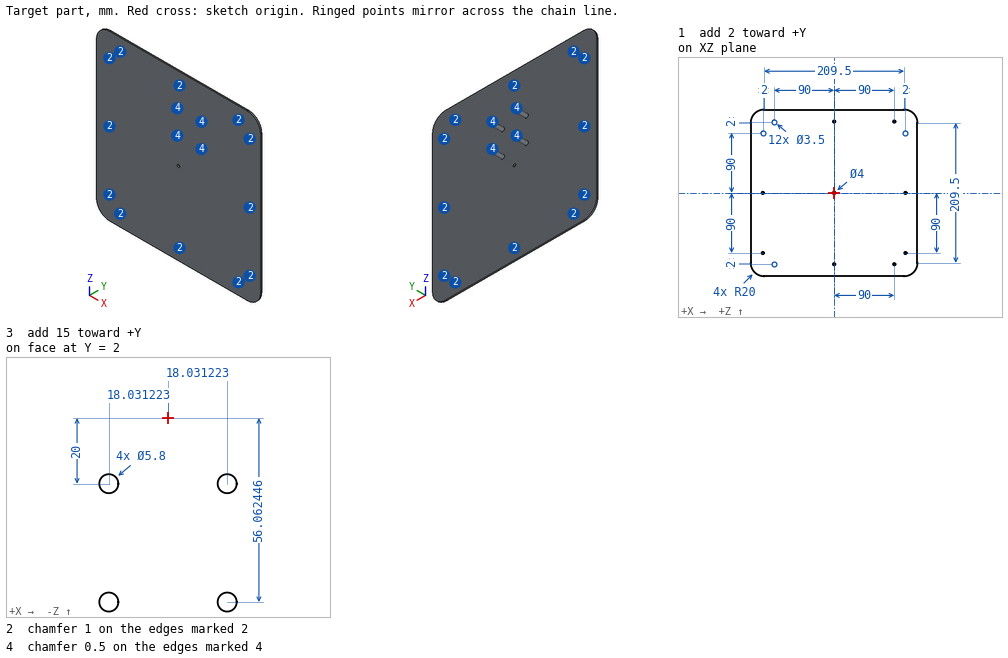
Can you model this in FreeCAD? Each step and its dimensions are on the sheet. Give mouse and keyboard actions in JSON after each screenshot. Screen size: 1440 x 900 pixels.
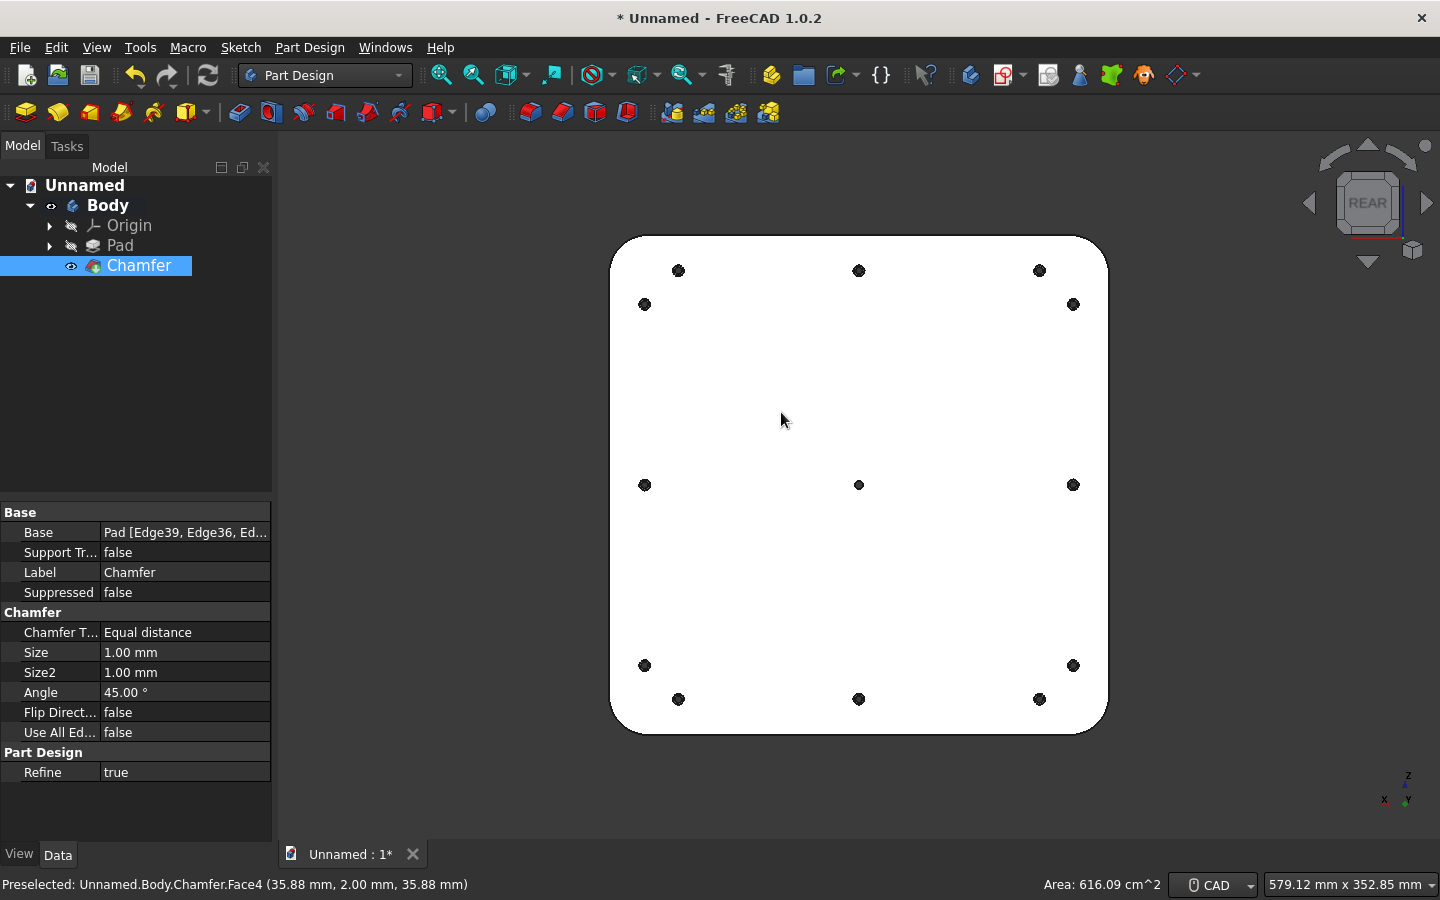
{"action": "left_click", "coordinate": [1004, 76]}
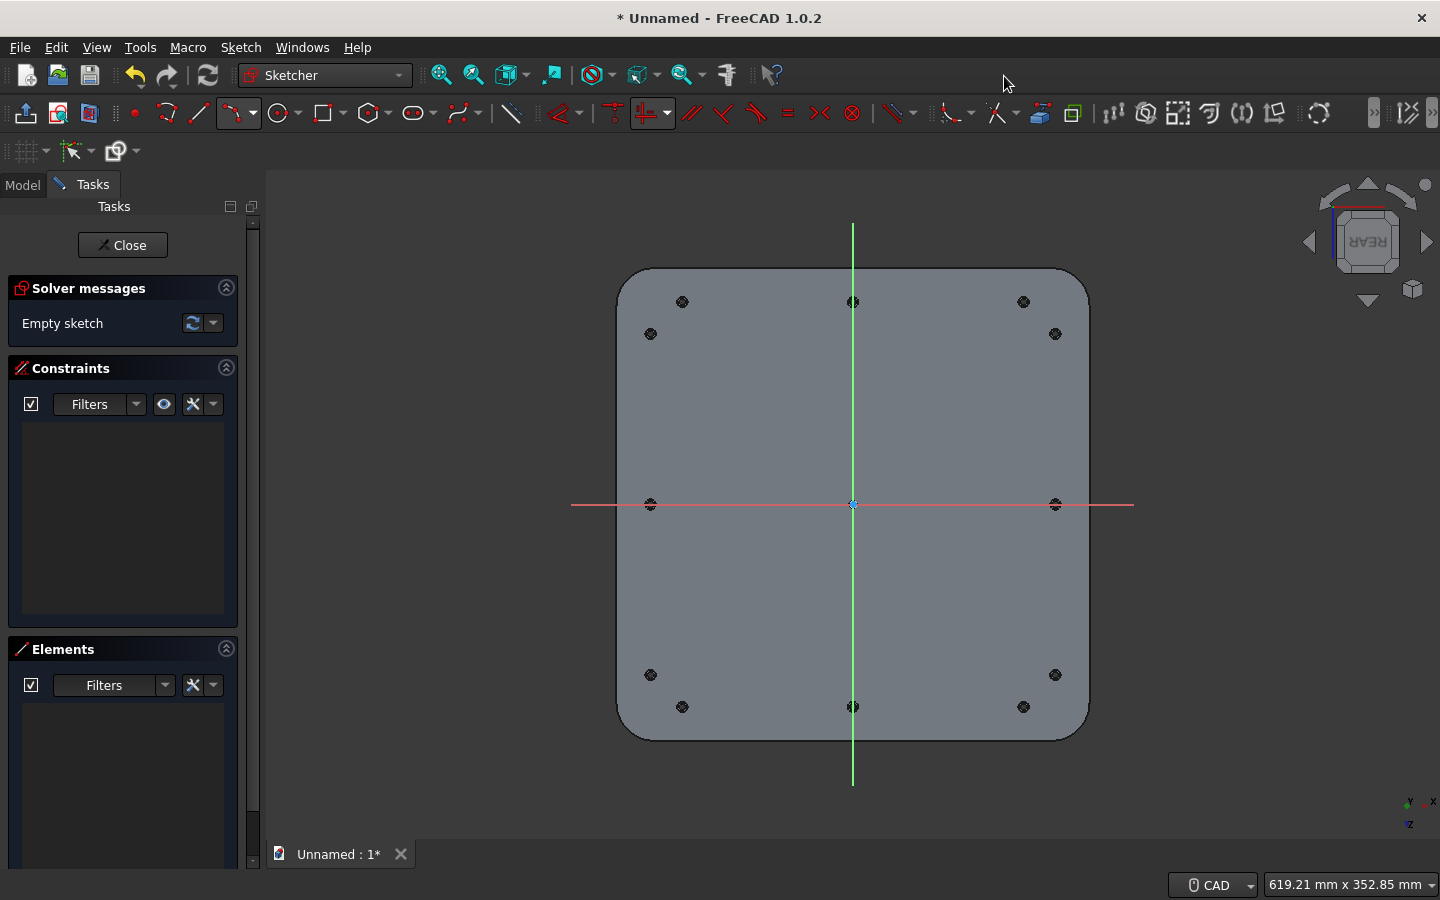
{"action": "scroll", "coordinate": [875, 579], "scroll_direction": "up", "scroll_amount": 7}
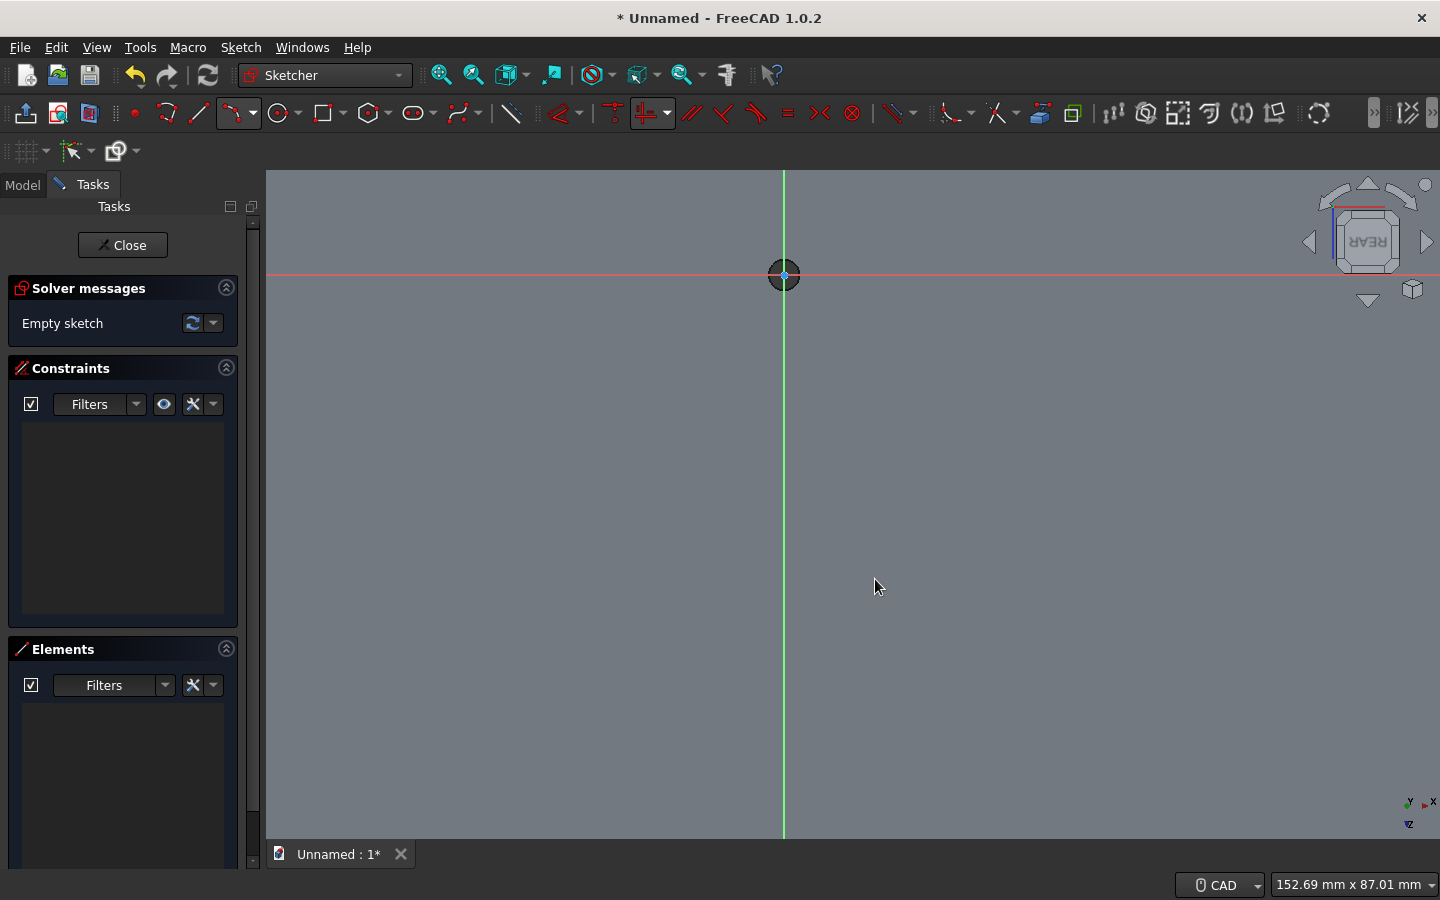
{"action": "key", "text": "g c"}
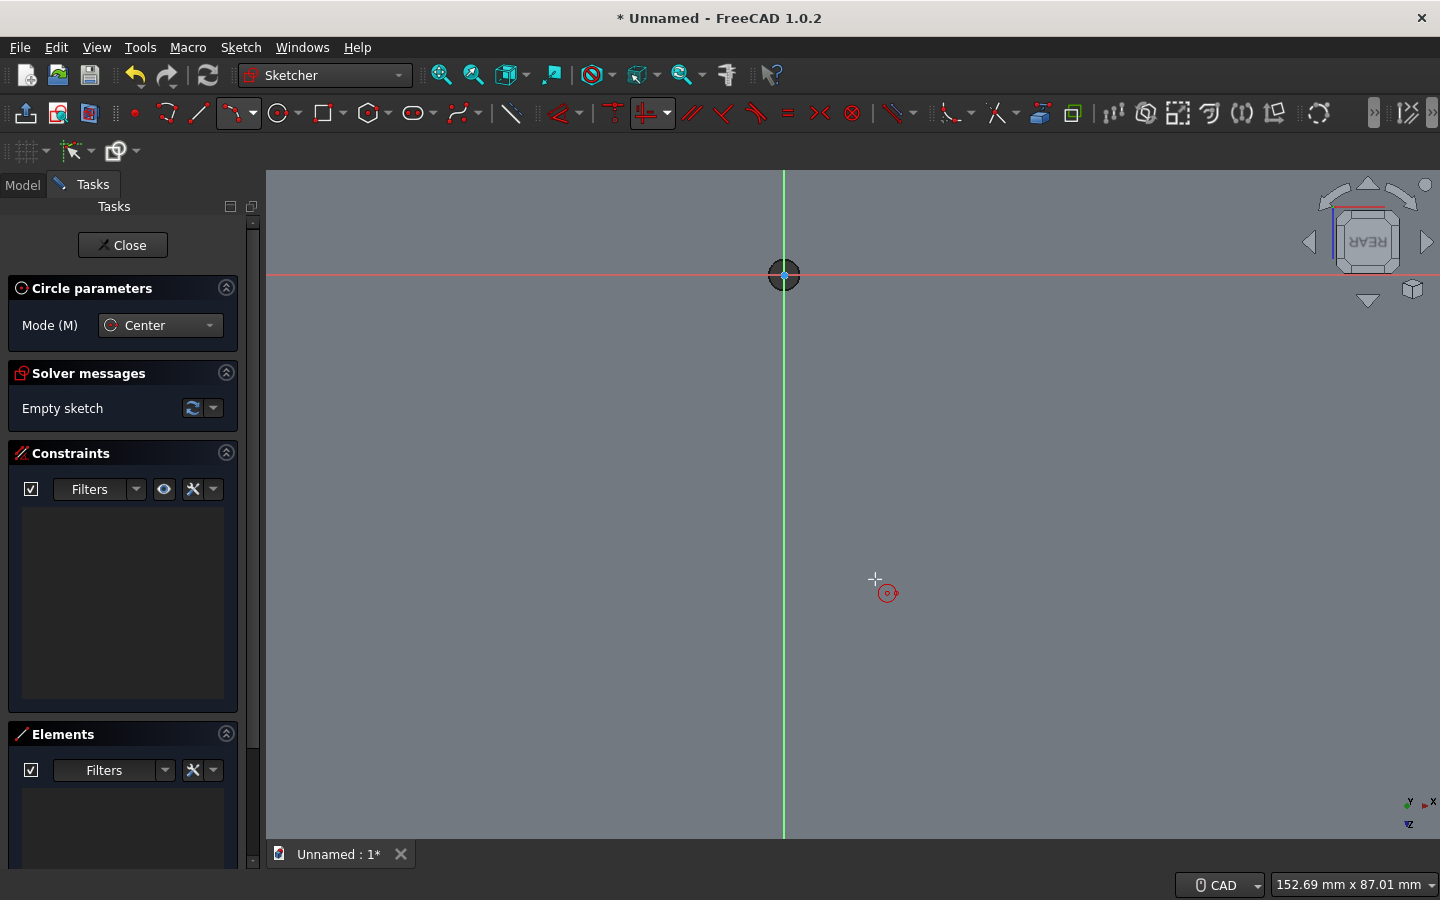
{"action": "left_click", "coordinate": [646, 429]}
{"action": "mouse_move", "coordinate": [661, 413]}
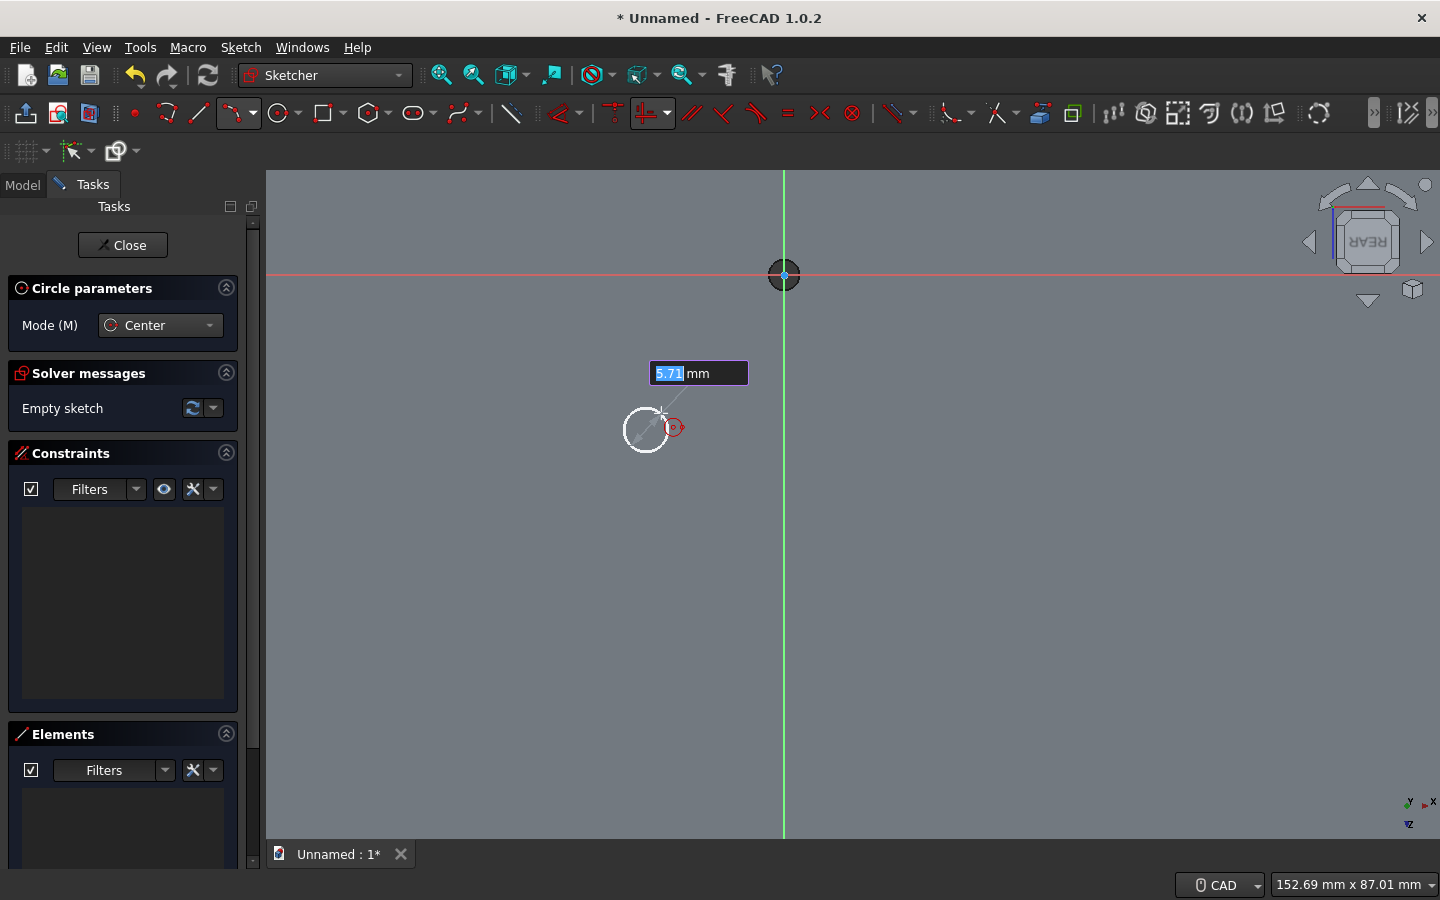
{"action": "type", "text": "5.8"}
{"action": "key", "text": "Return"}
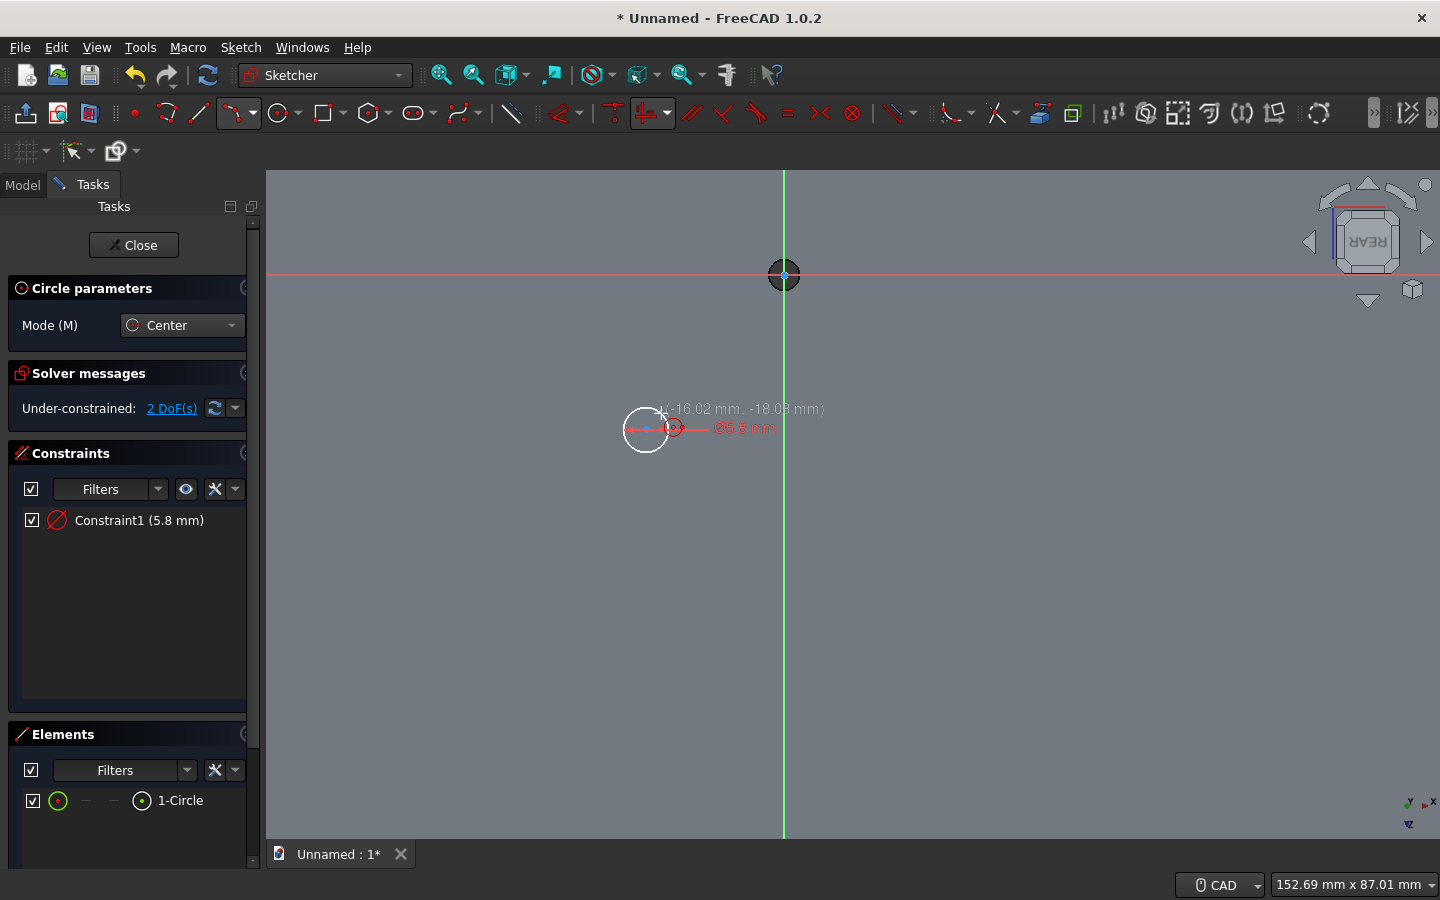
{"action": "left_click", "coordinate": [923, 429]}
{"action": "mouse_move", "coordinate": [939, 413]}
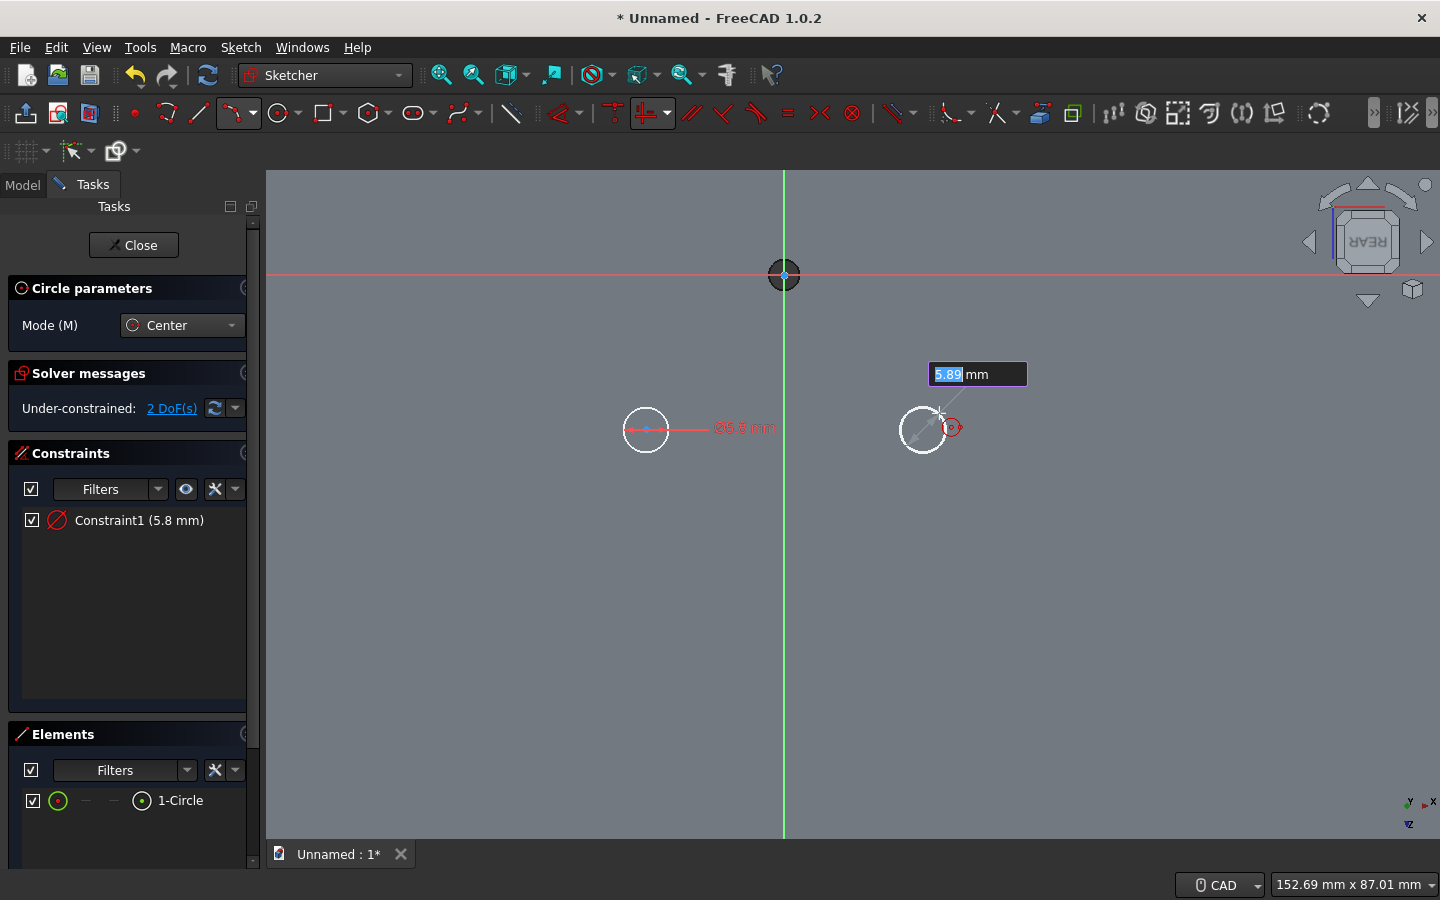
{"action": "type", "text": "5.8"}
{"action": "key", "text": "Return"}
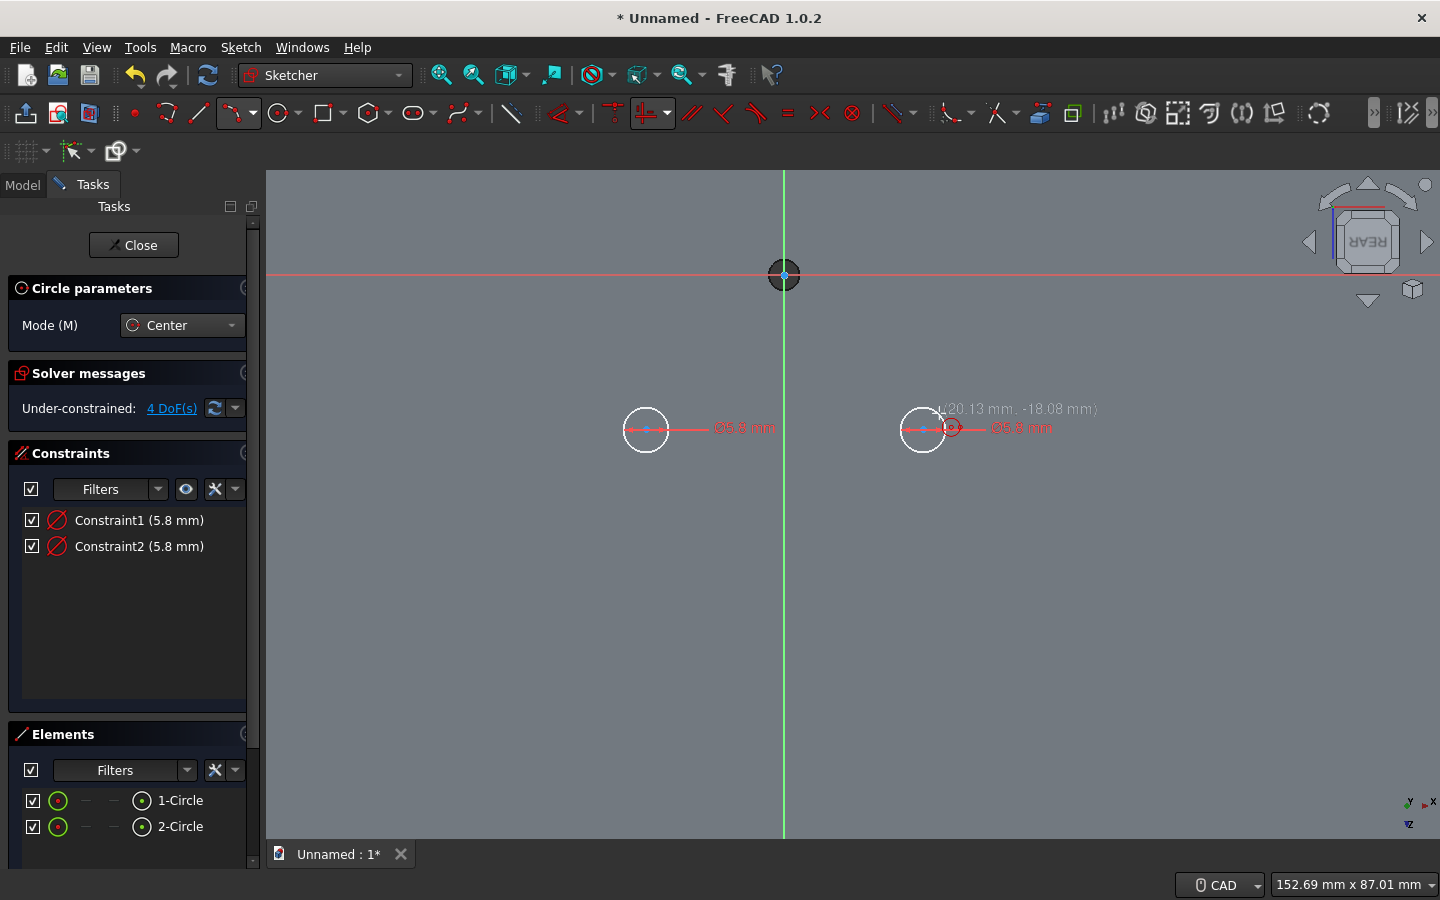
{"action": "left_click", "coordinate": [923, 706]}
{"action": "mouse_move", "coordinate": [939, 690]}